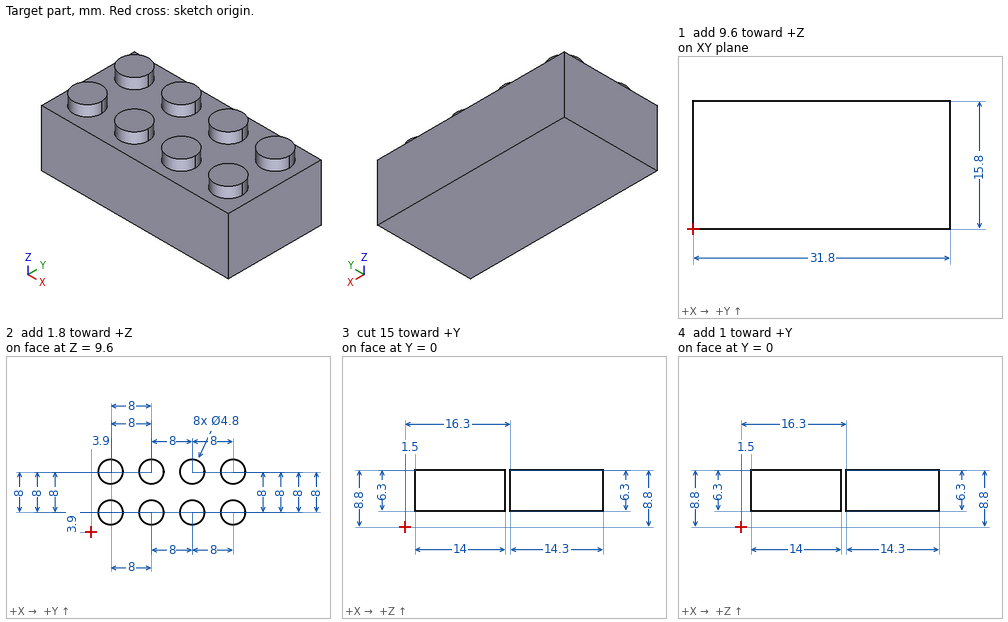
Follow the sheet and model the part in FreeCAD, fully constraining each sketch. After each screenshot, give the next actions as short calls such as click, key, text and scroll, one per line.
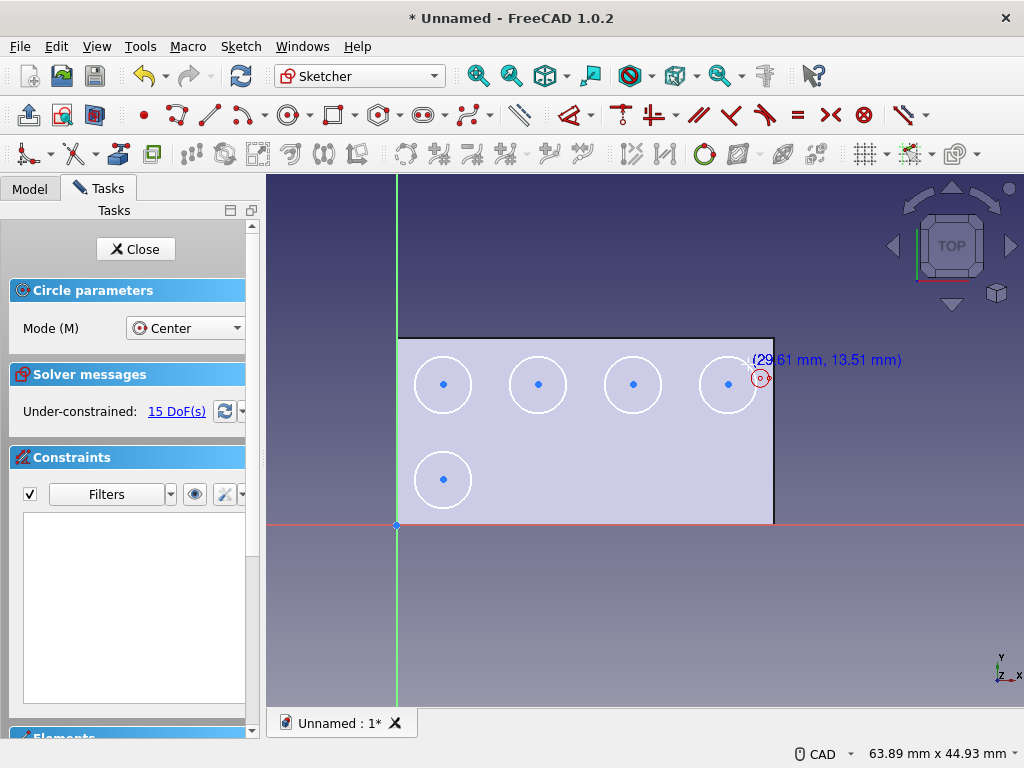
click(538, 479)
click(558, 459)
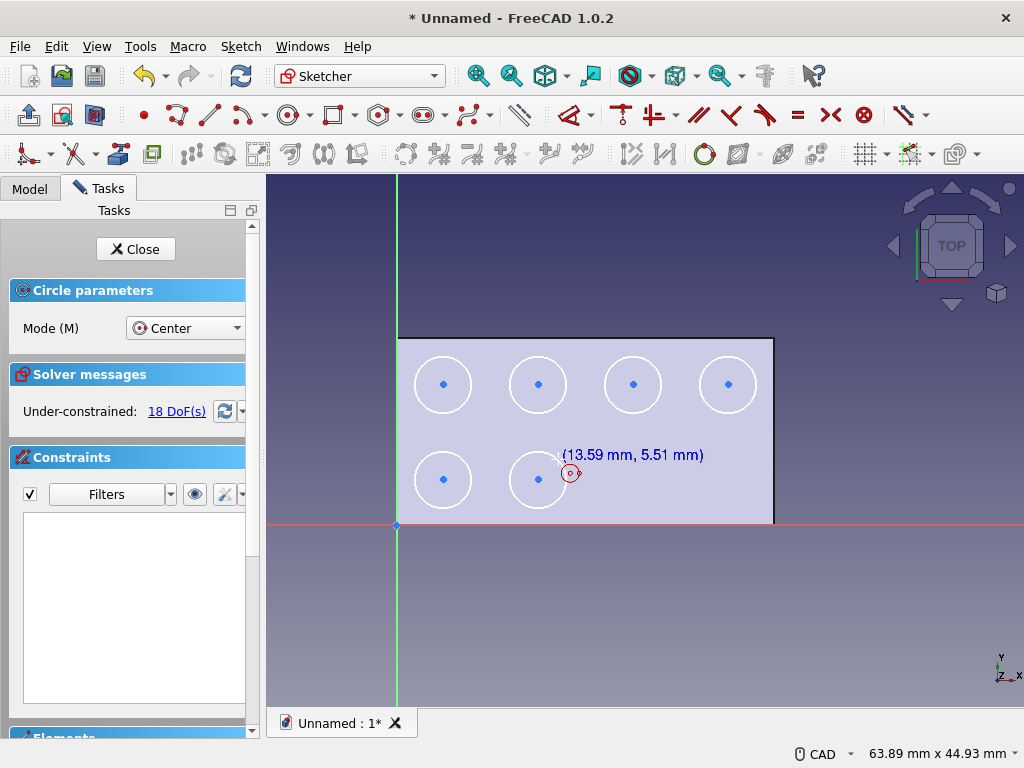
click(633, 479)
click(653, 459)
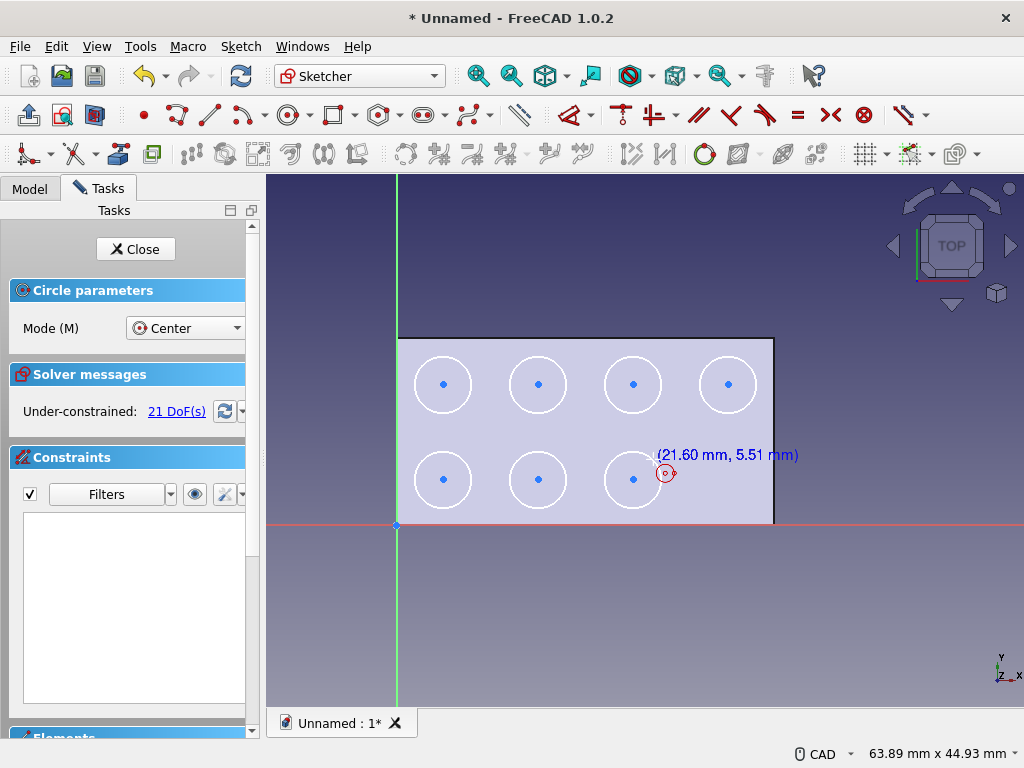
click(728, 479)
click(748, 459)
key(Escape)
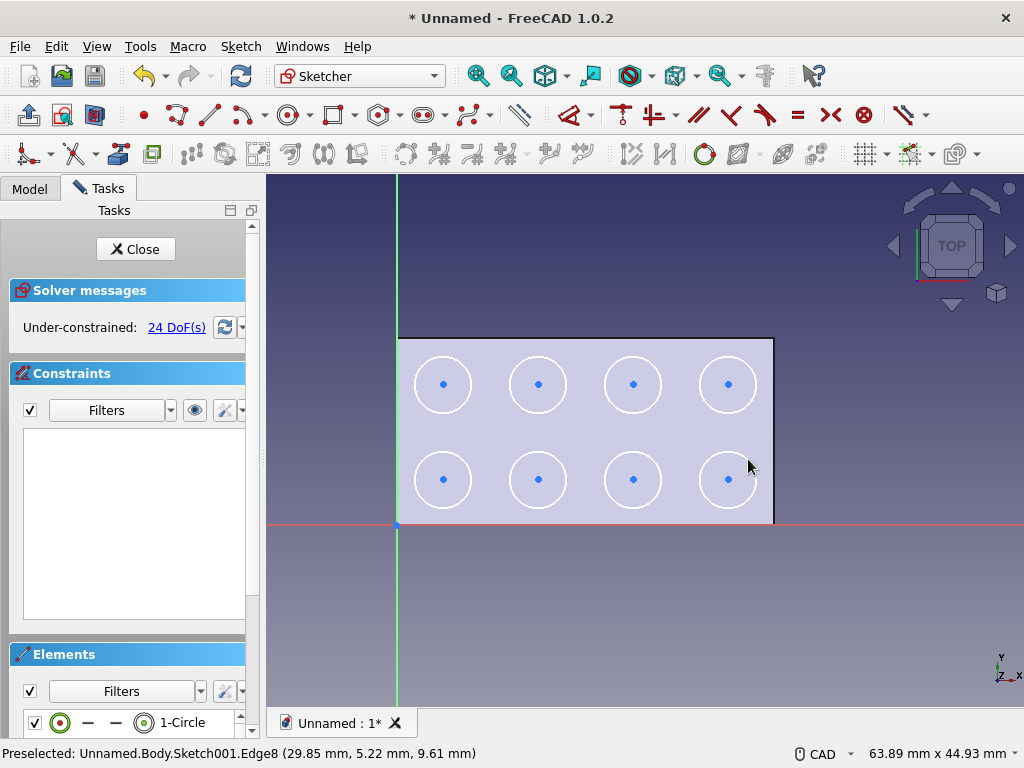
click(463, 365)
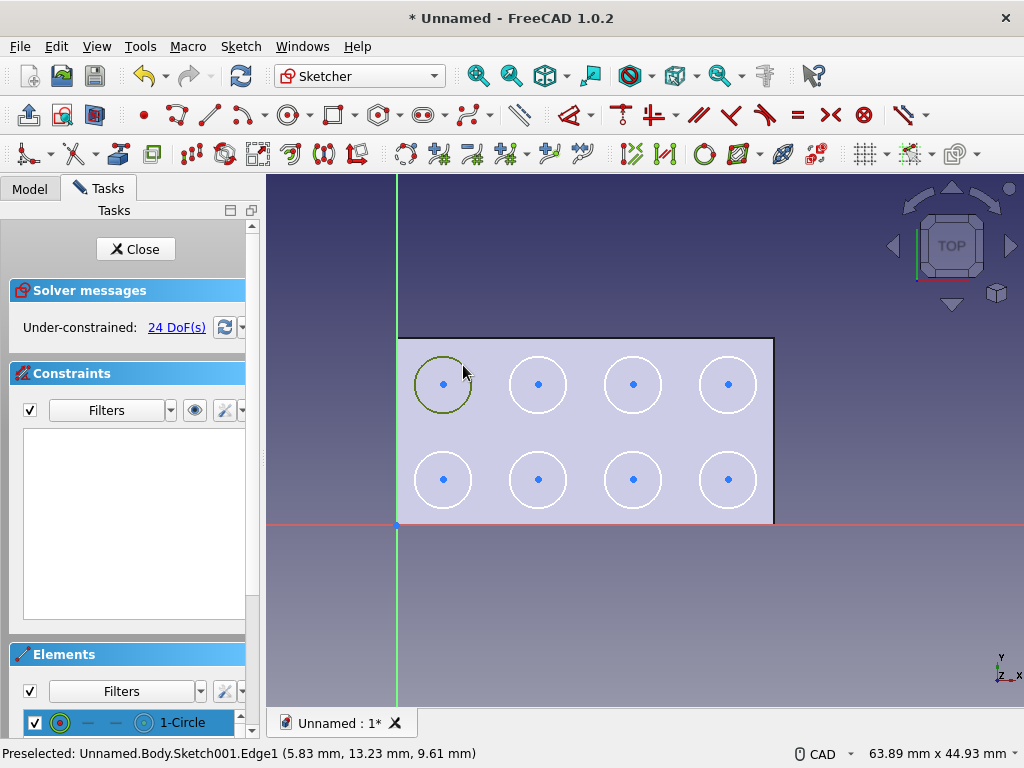
click(463, 460)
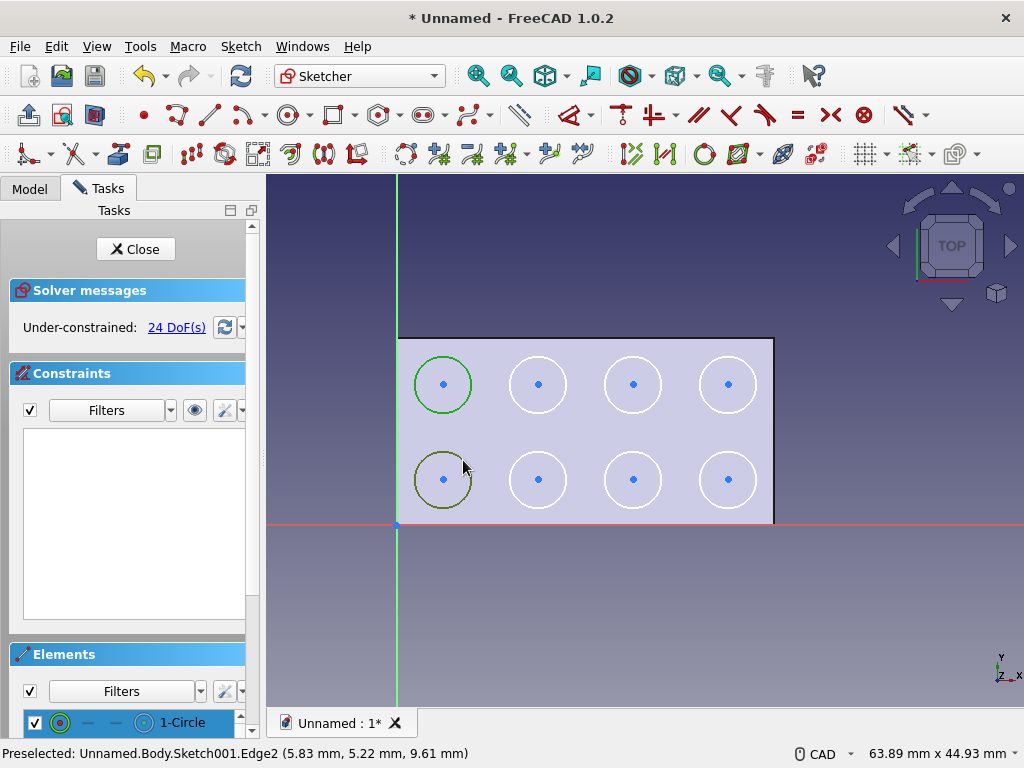
click(558, 365)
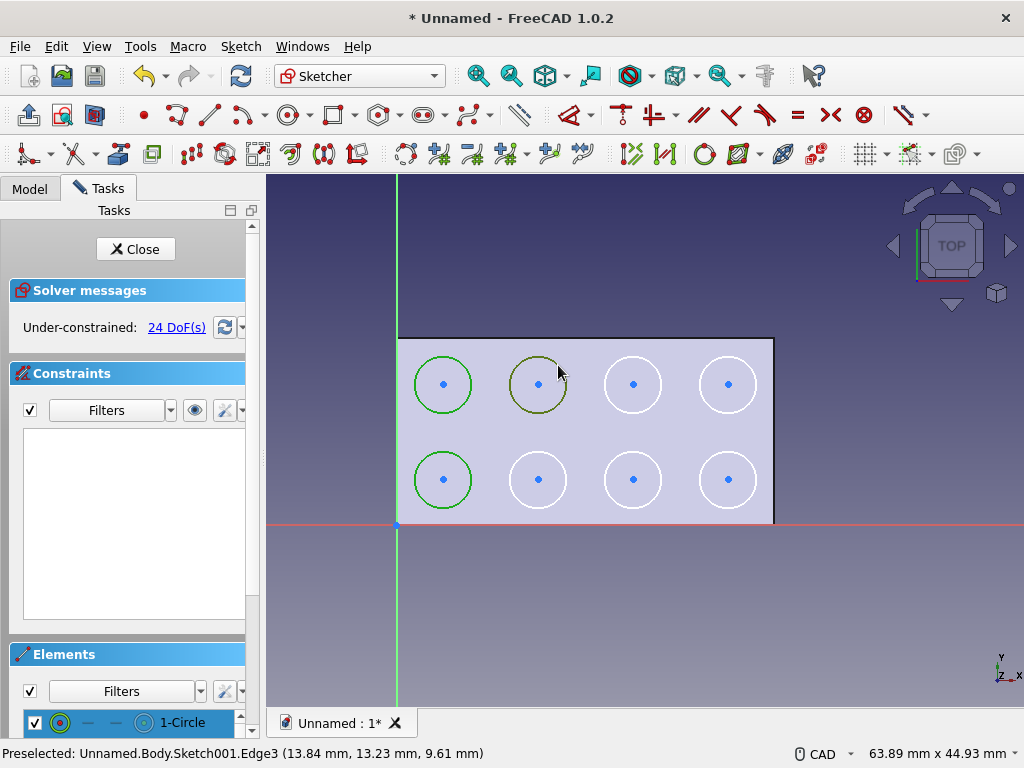
click(653, 365)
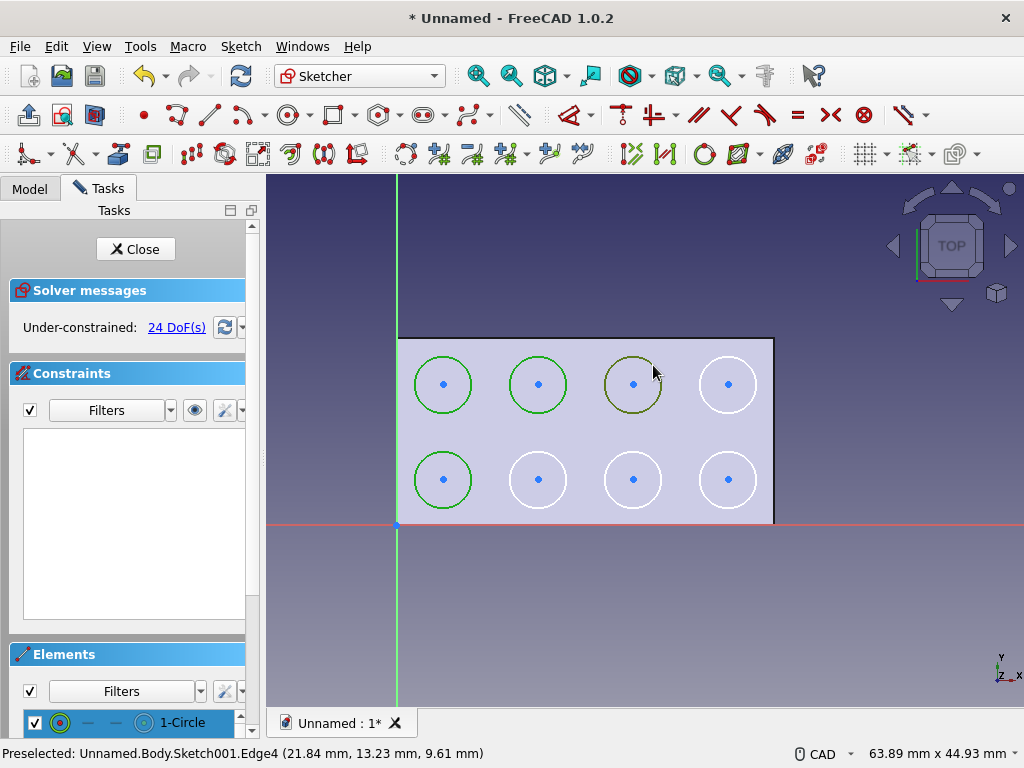
click(748, 365)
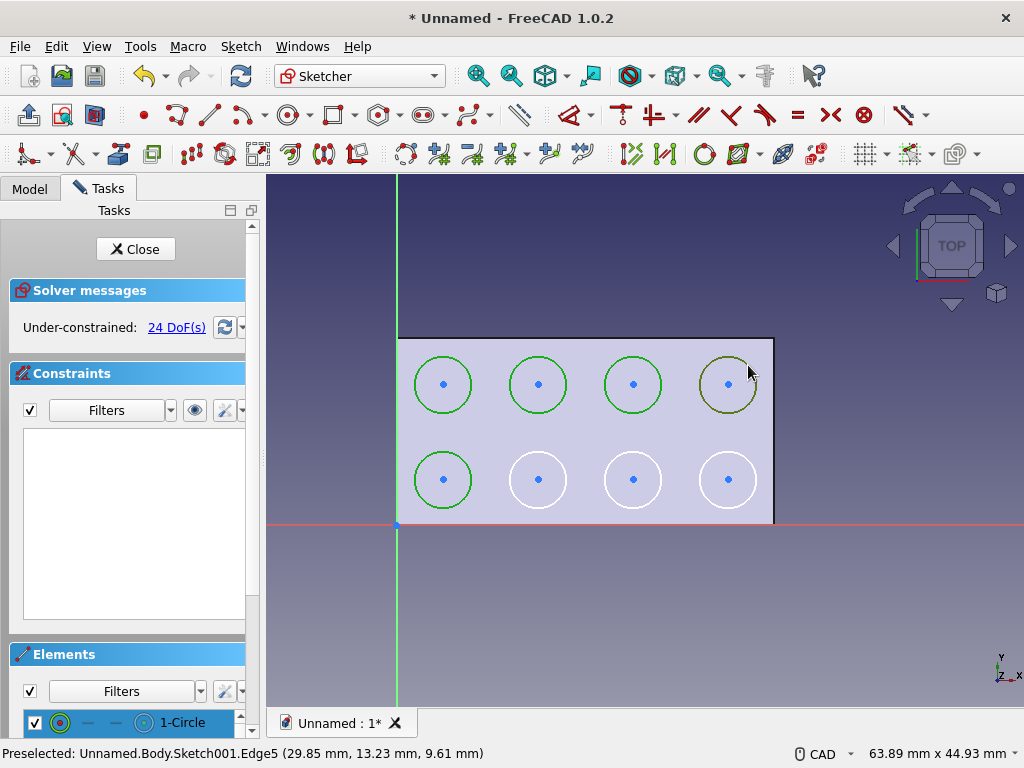
click(558, 460)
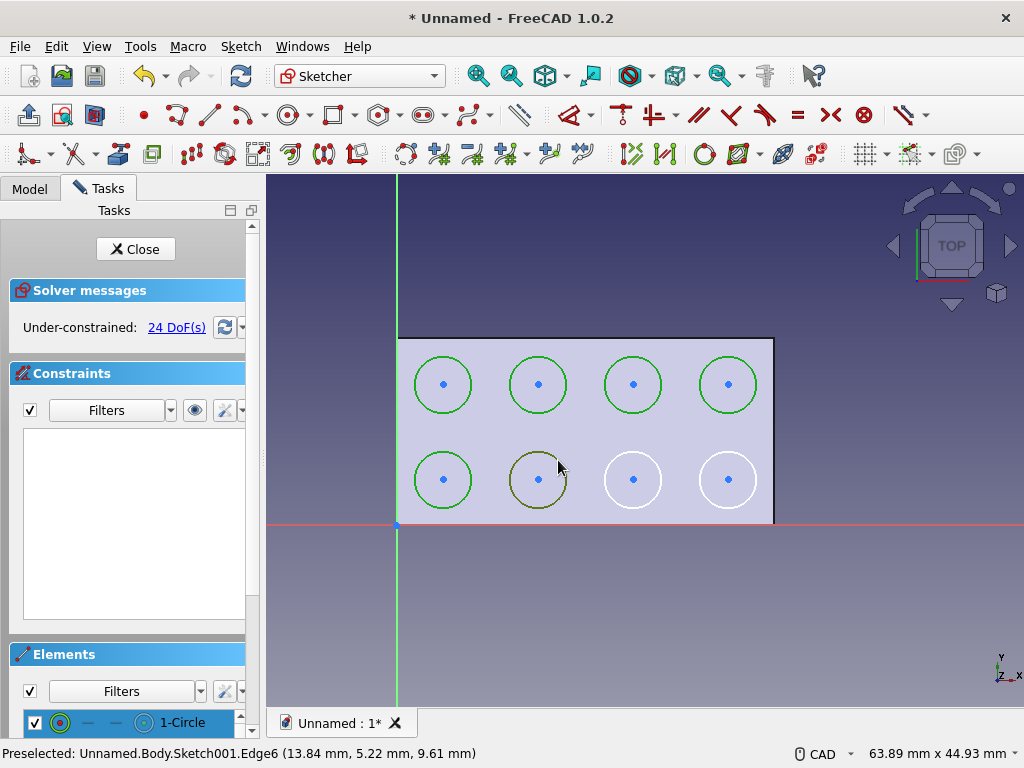
click(653, 460)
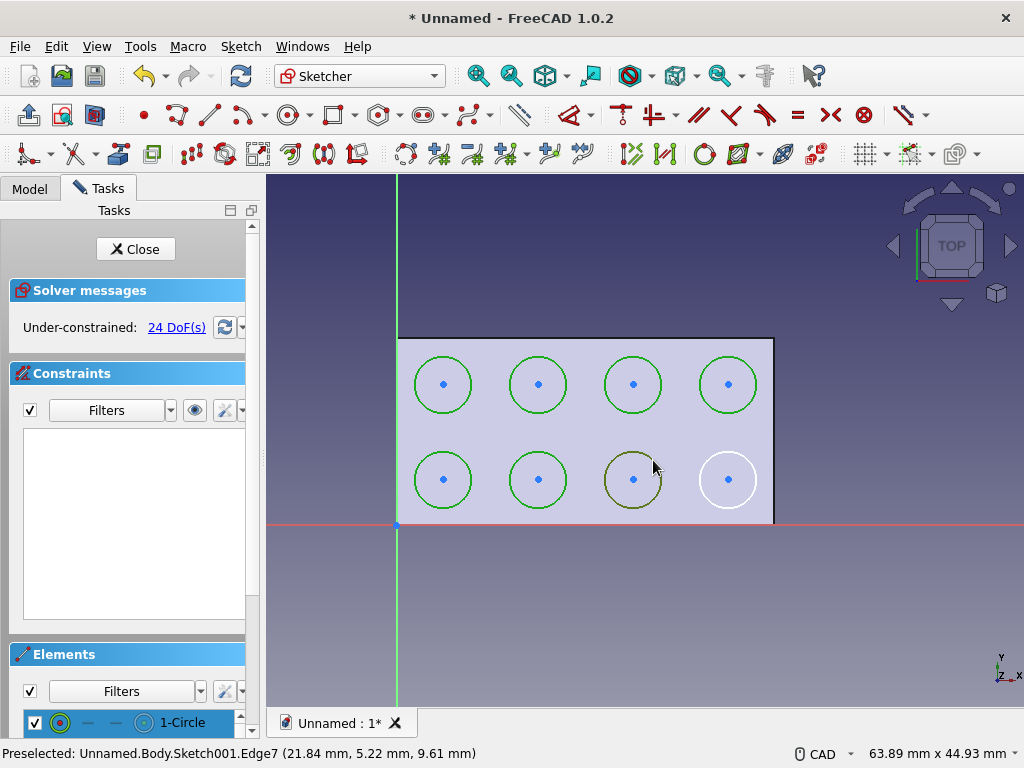
click(748, 460)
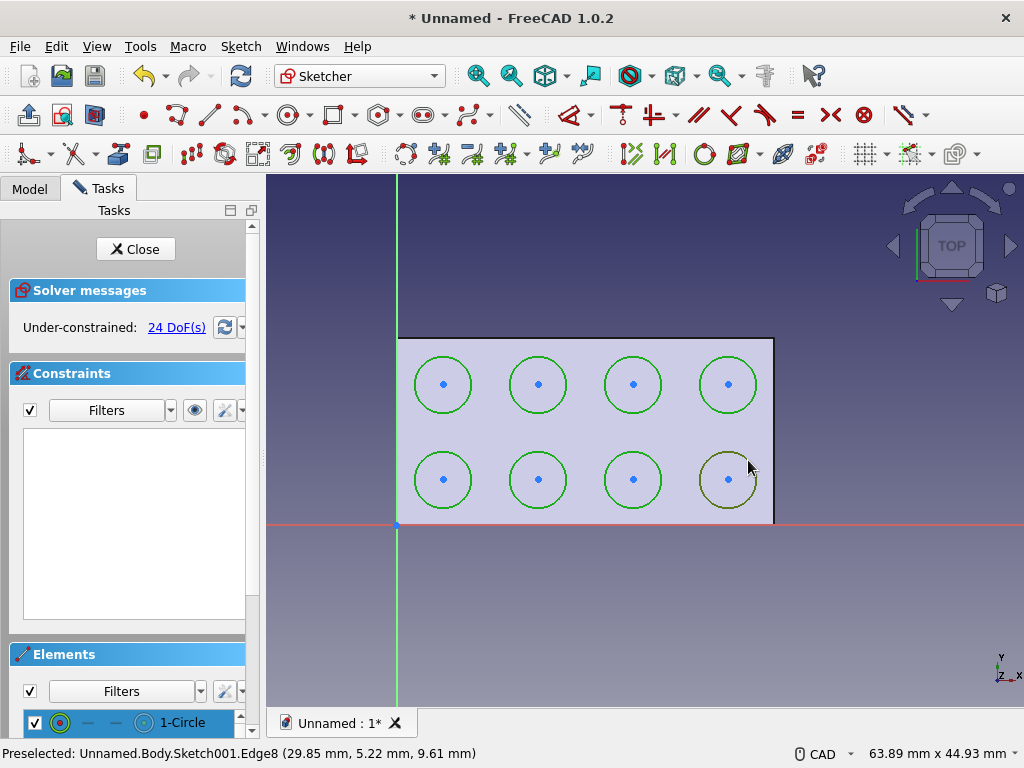
click(798, 116)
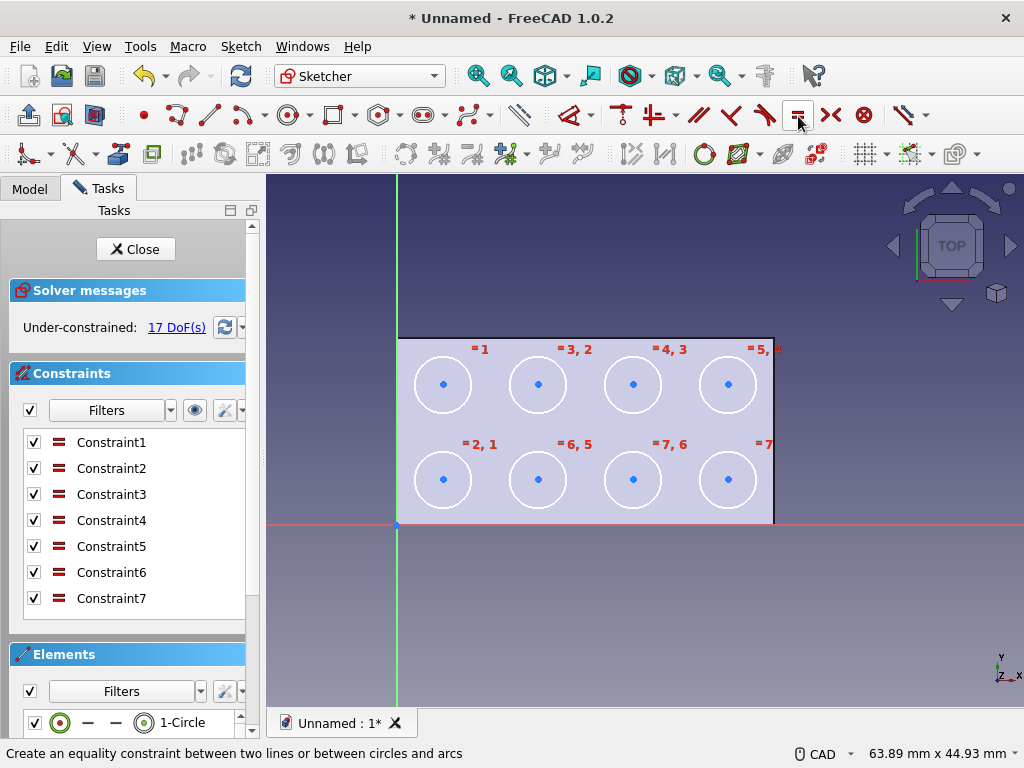
key(d)